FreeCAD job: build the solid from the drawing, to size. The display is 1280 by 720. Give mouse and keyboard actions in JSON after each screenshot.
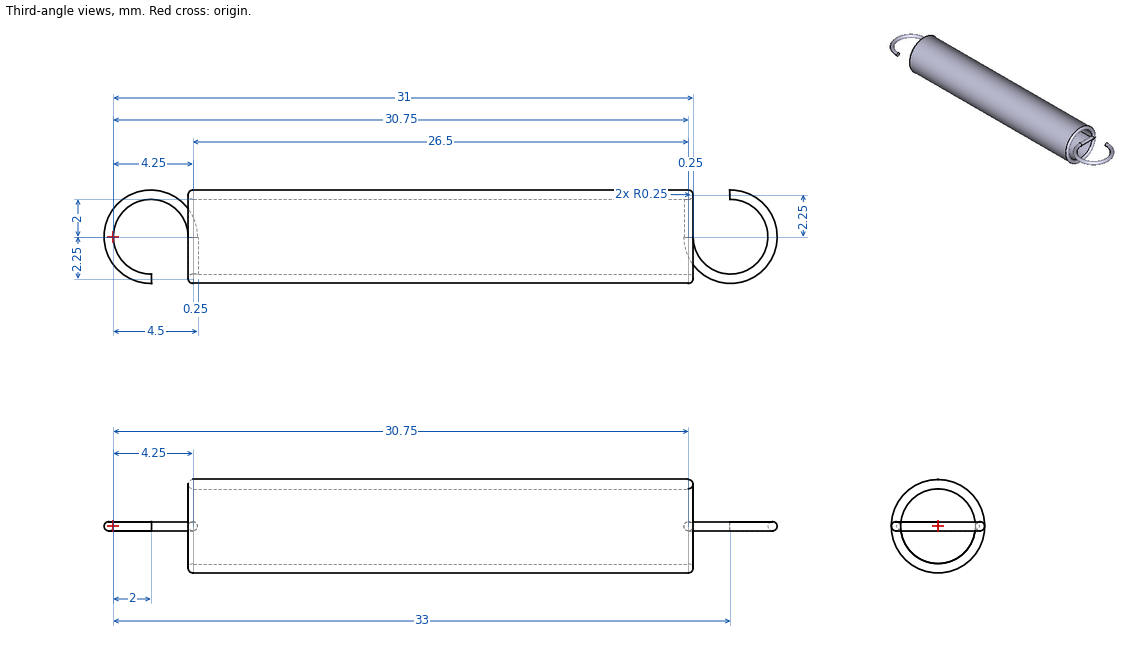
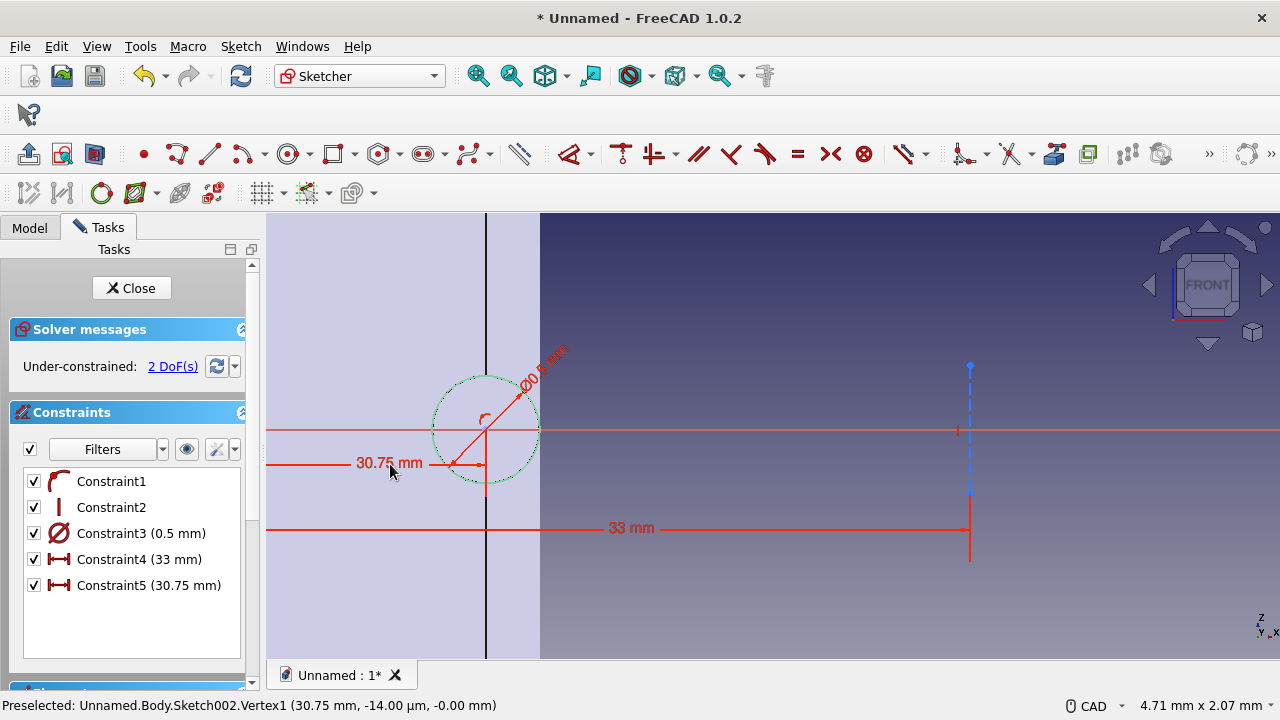
{"action": "left_click", "coordinate": [132, 288]}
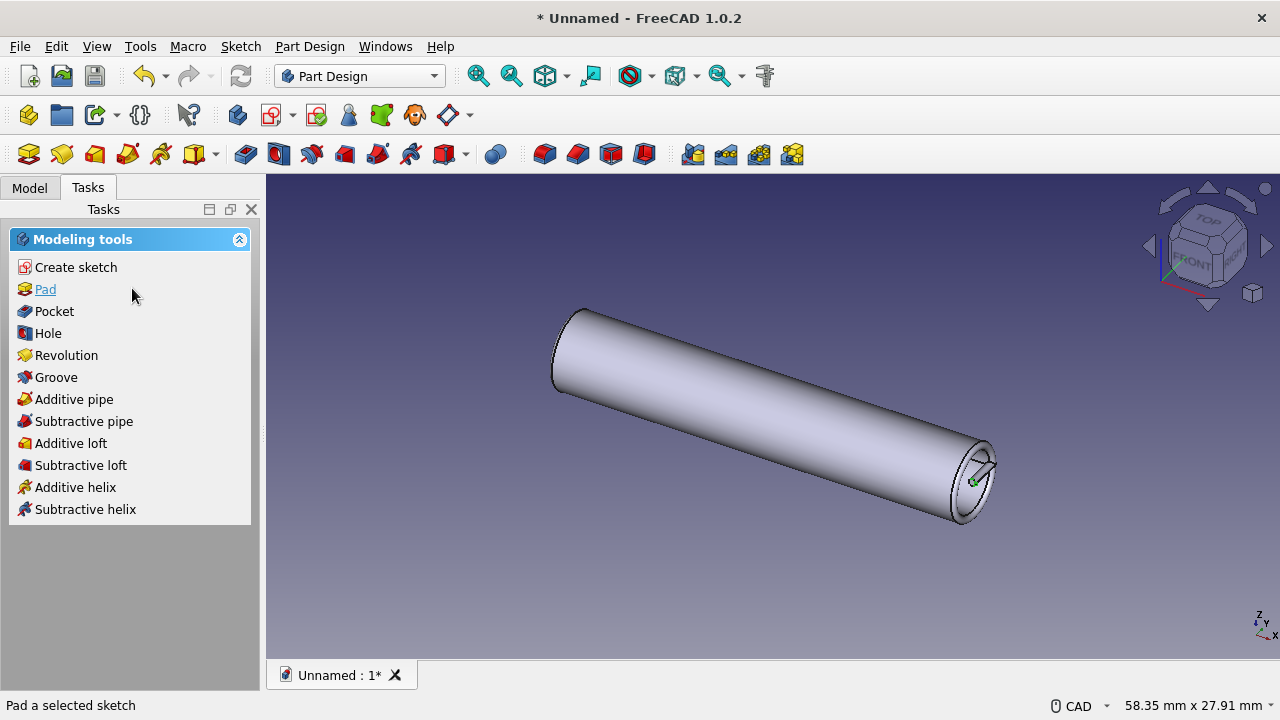
{"action": "left_click", "coordinate": [62, 154]}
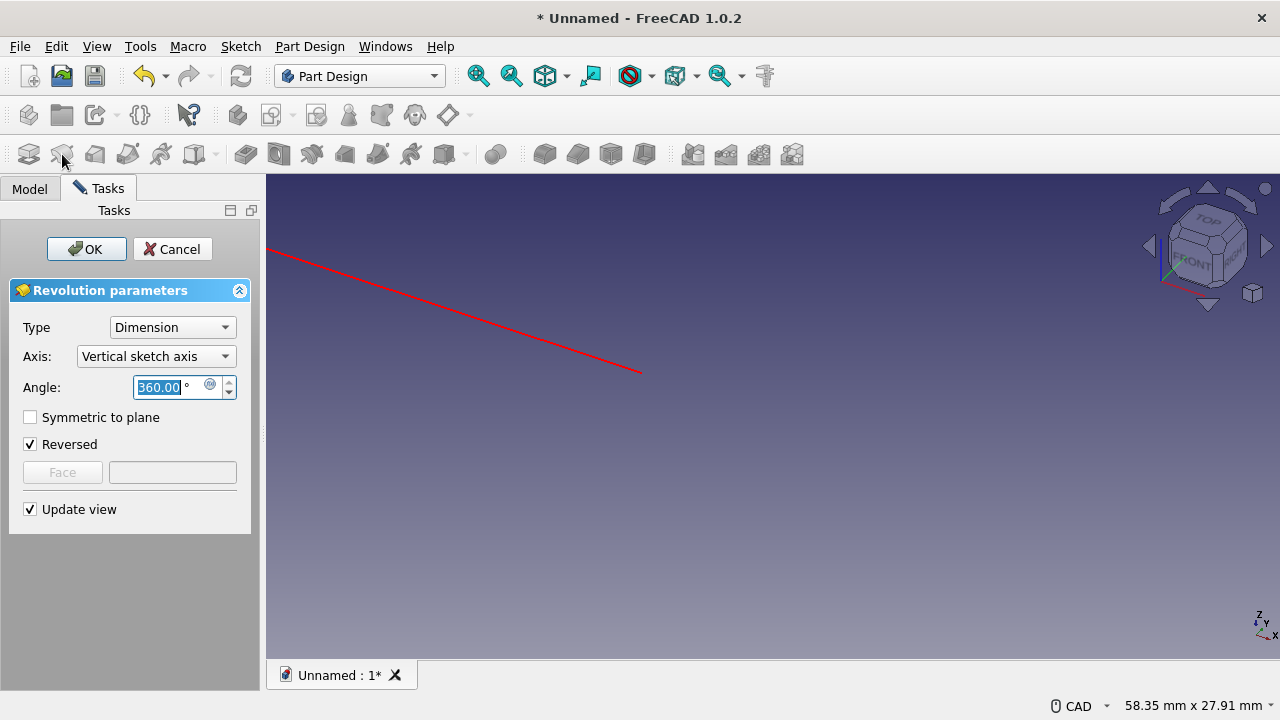
{"action": "left_click", "coordinate": [157, 356]}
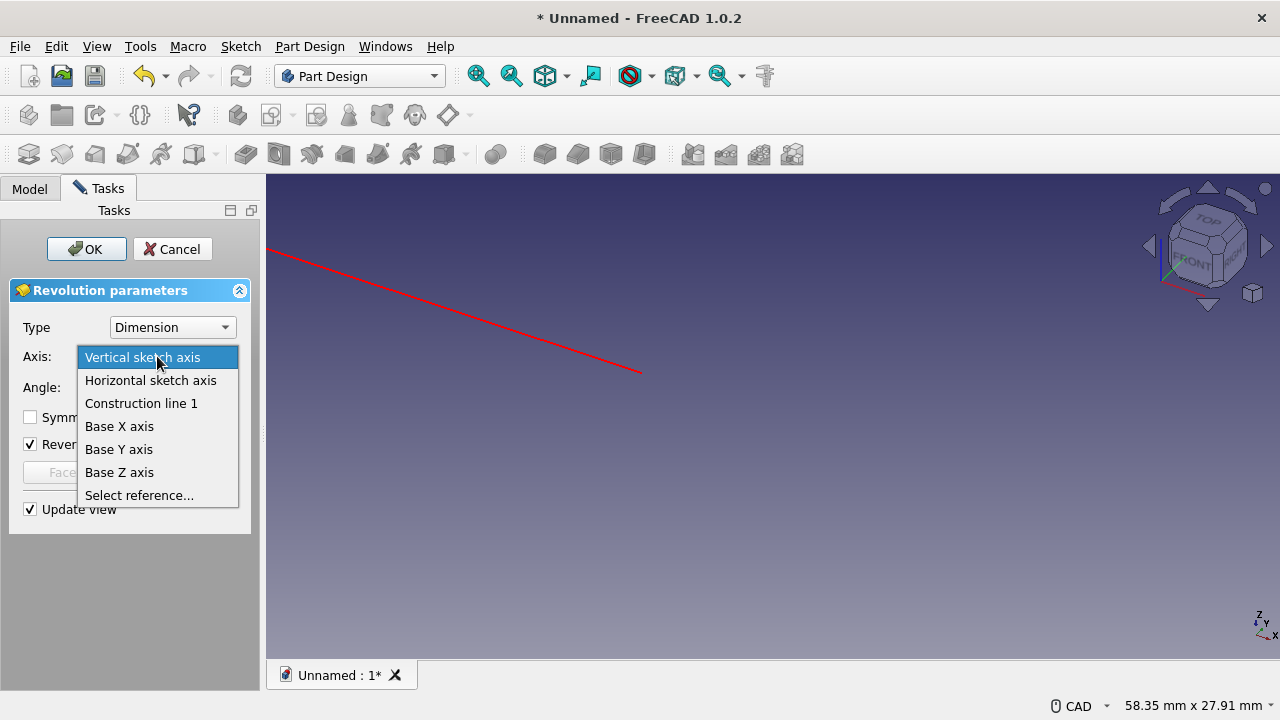
{"action": "left_click", "coordinate": [156, 404]}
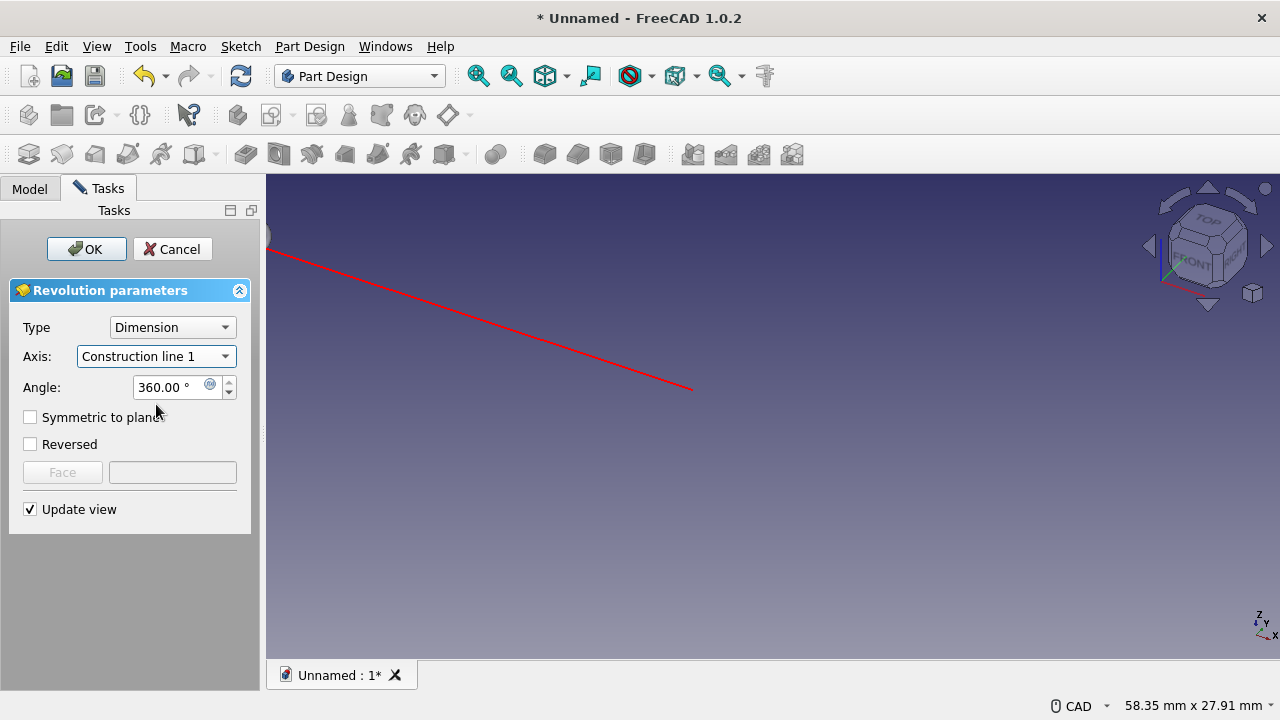
{"action": "triple_click", "coordinate": [178, 388]}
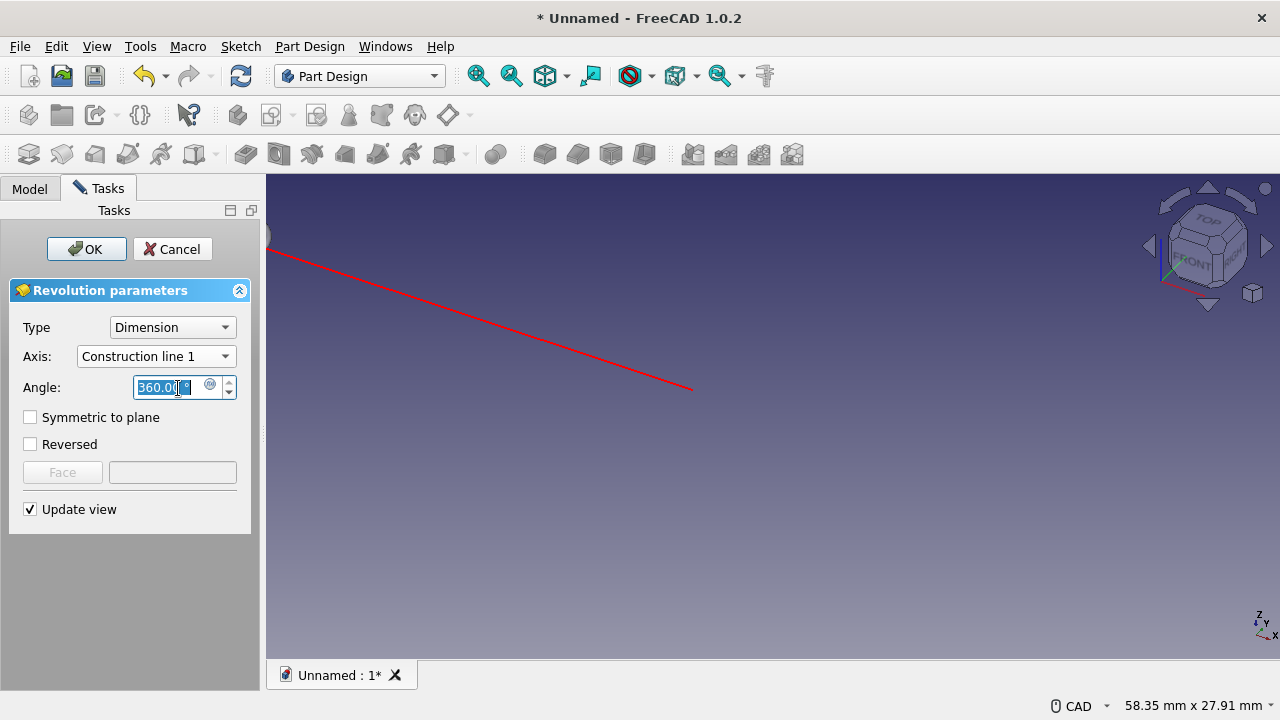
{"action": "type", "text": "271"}
{"action": "key", "text": "Tab"}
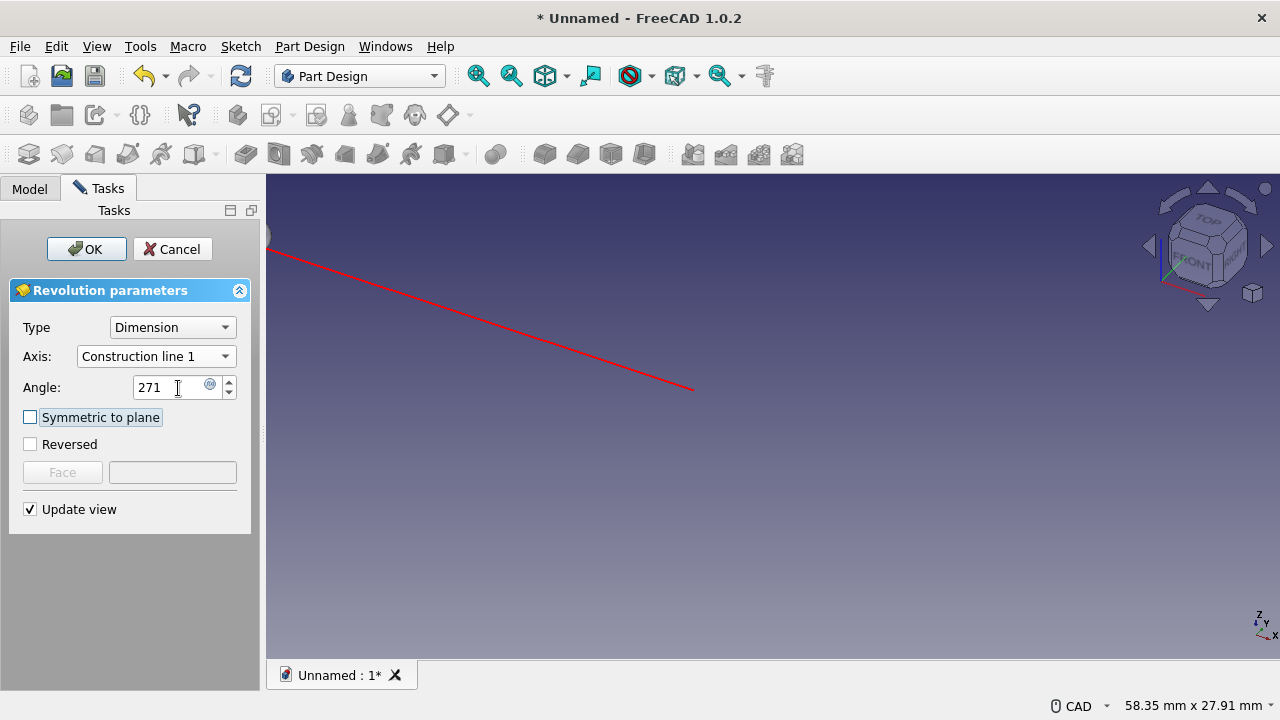
{"action": "left_click", "coordinate": [87, 249]}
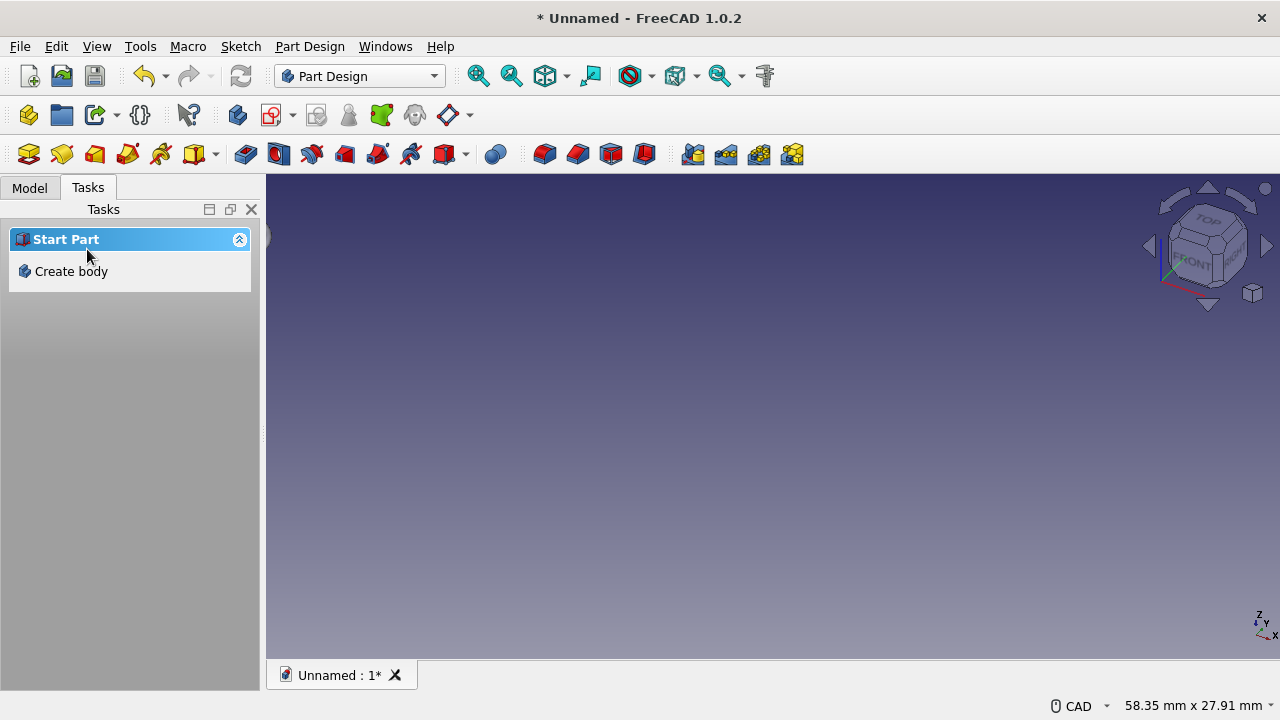
{"action": "left_click", "coordinate": [479, 76]}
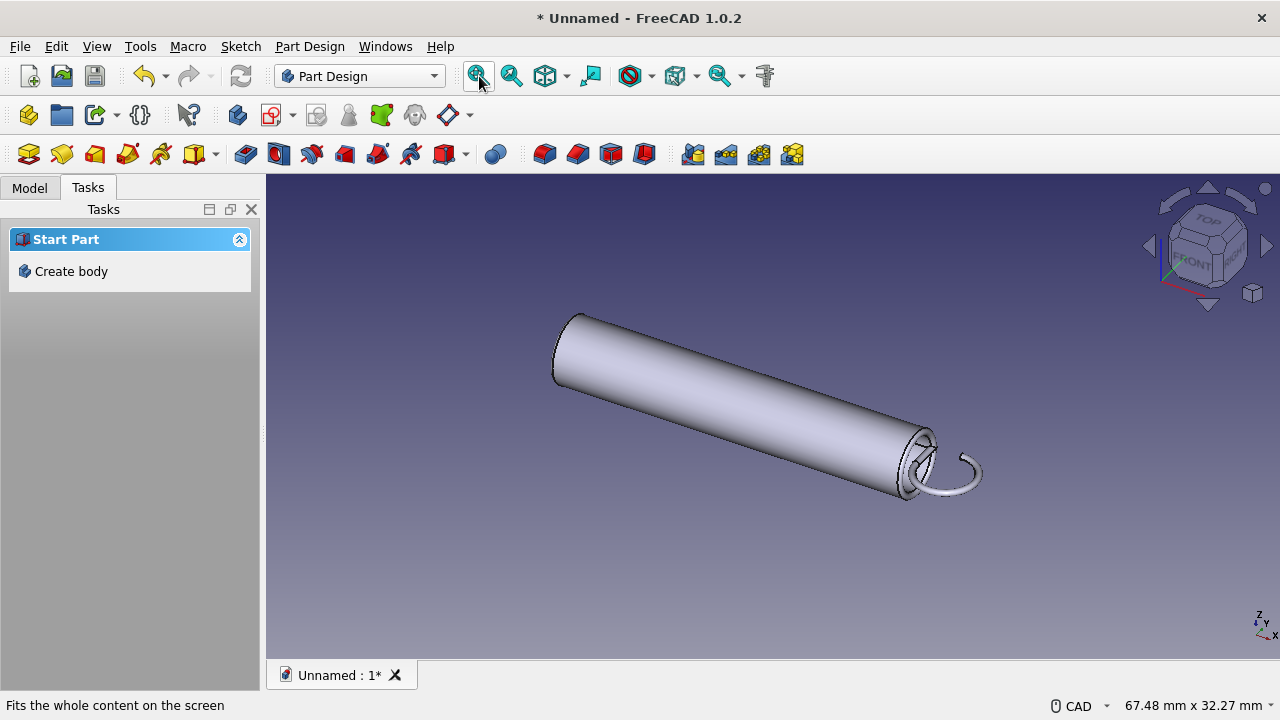
{"action": "left_click", "coordinate": [270, 116]}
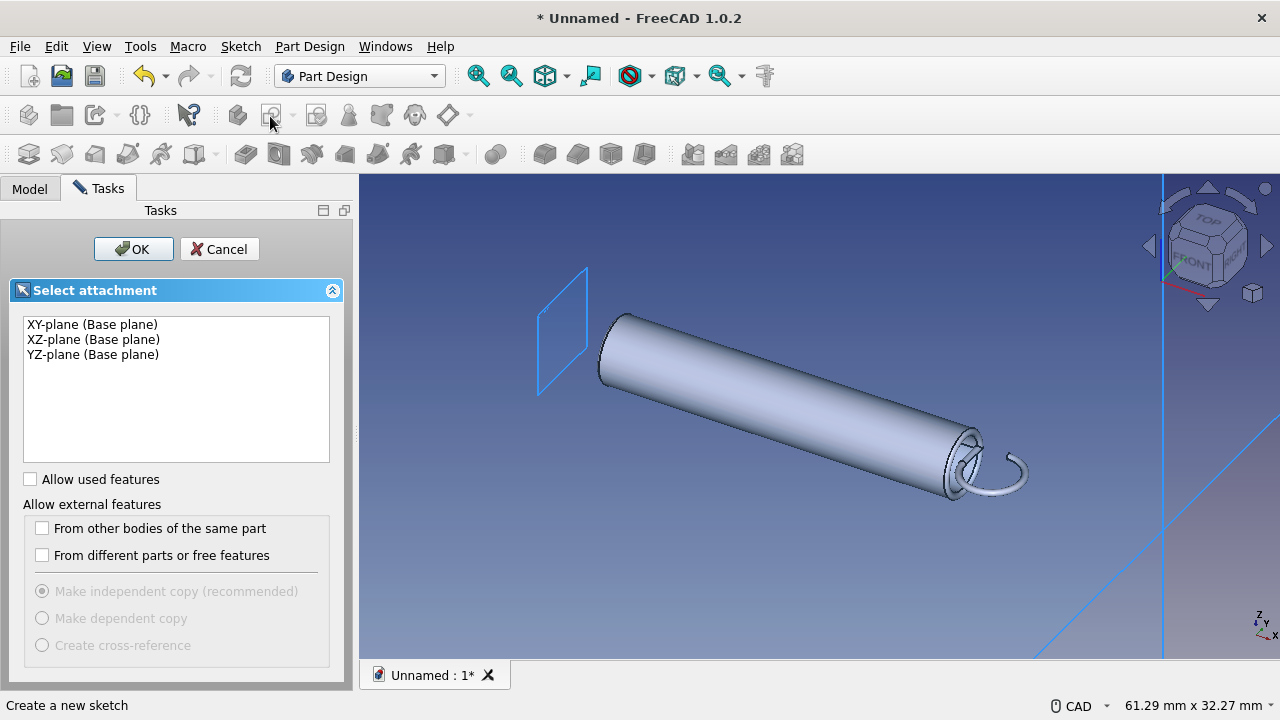
{"action": "left_click", "coordinate": [84, 324]}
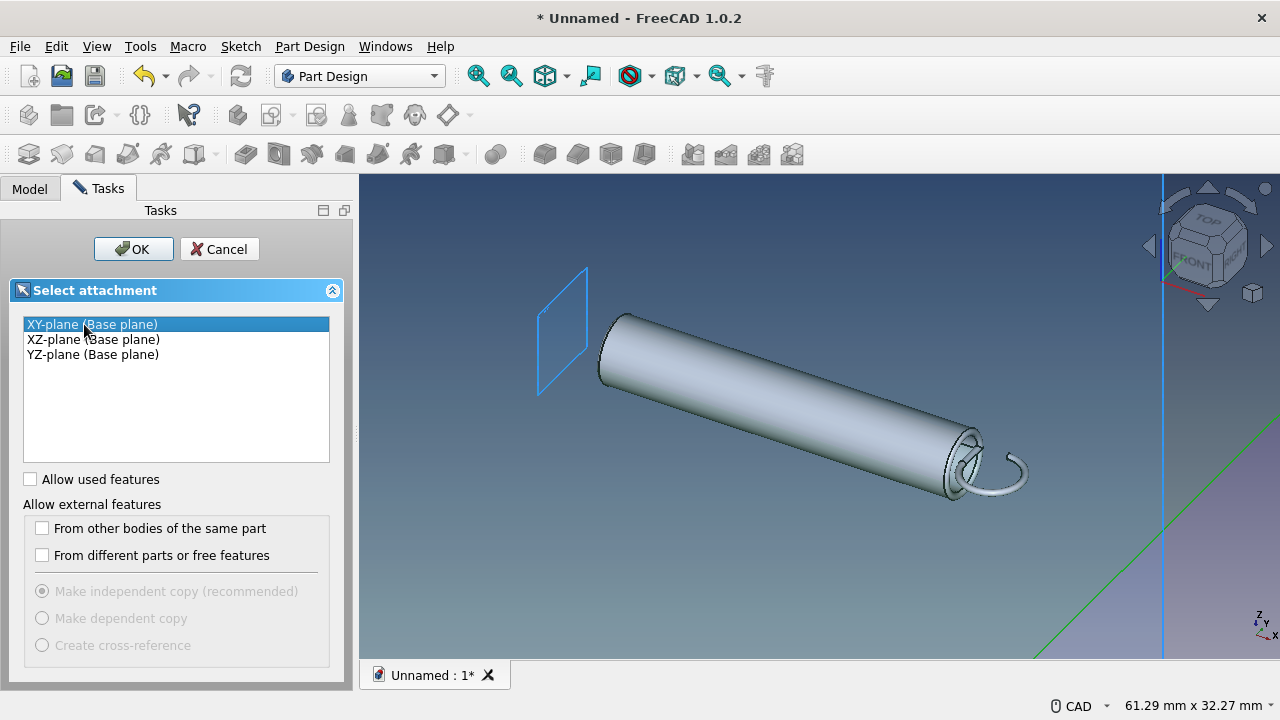
{"action": "left_click", "coordinate": [134, 249]}